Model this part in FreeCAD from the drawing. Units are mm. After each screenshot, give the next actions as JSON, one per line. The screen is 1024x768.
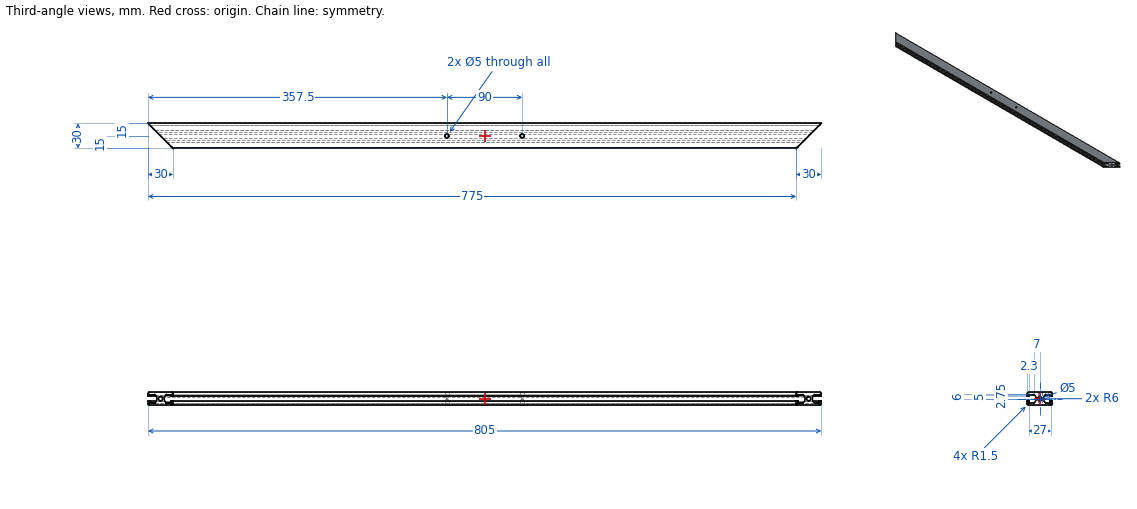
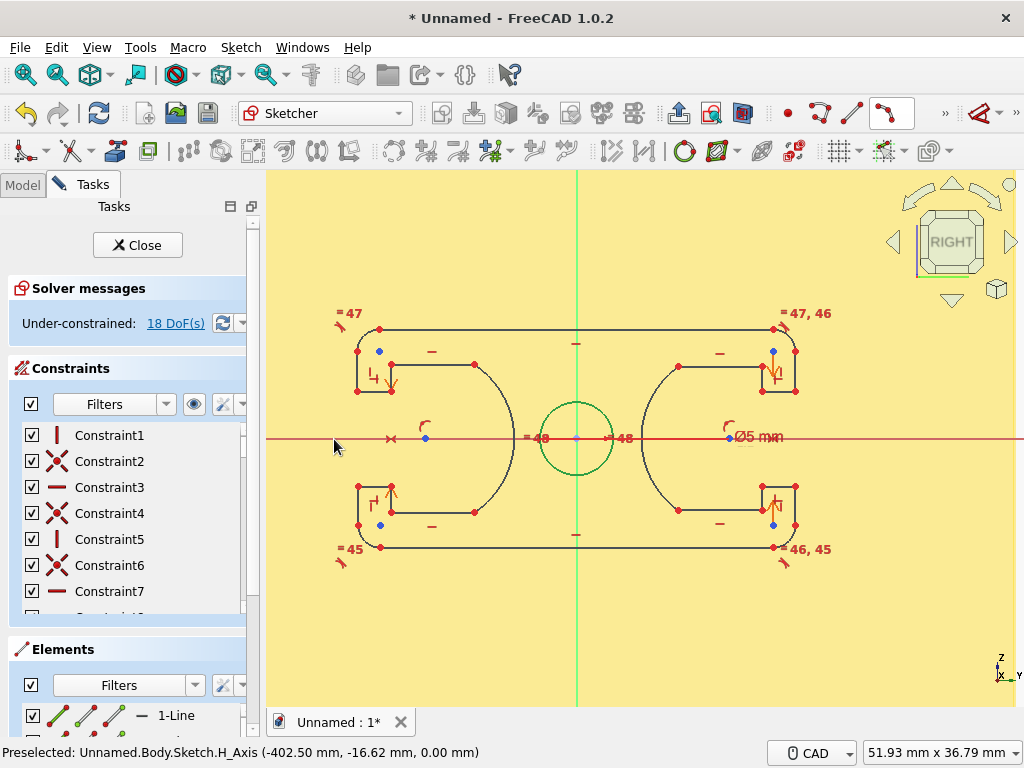
{"action": "left_click", "coordinate": [357, 392]}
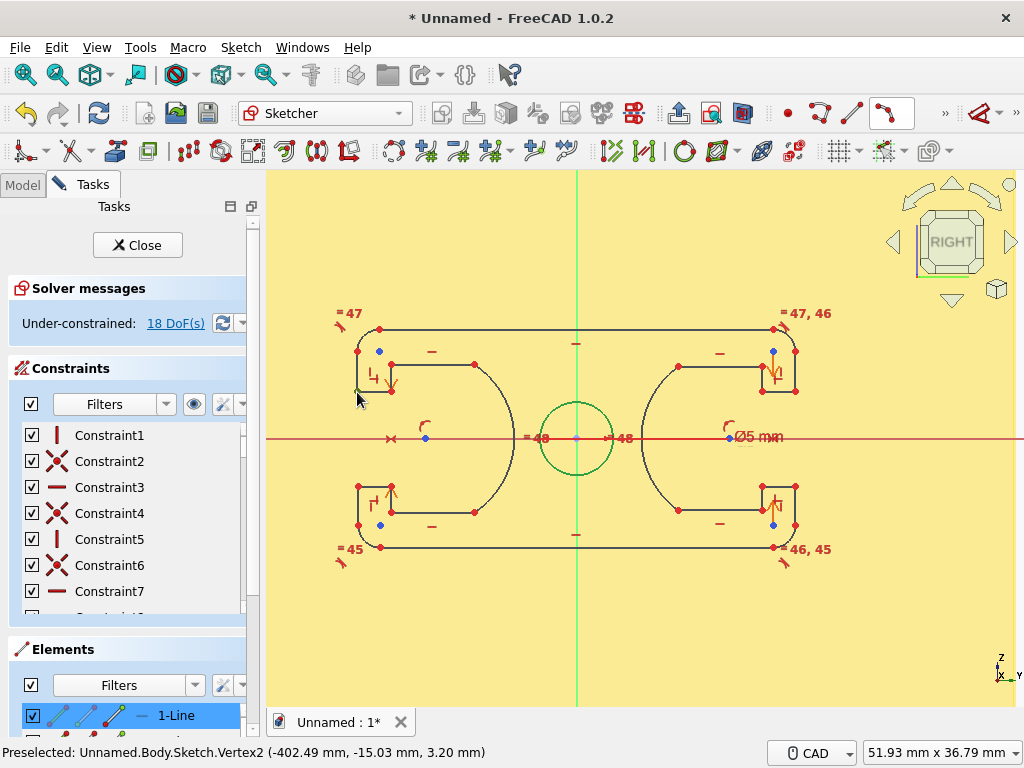
{"action": "left_click", "coordinate": [358, 487]}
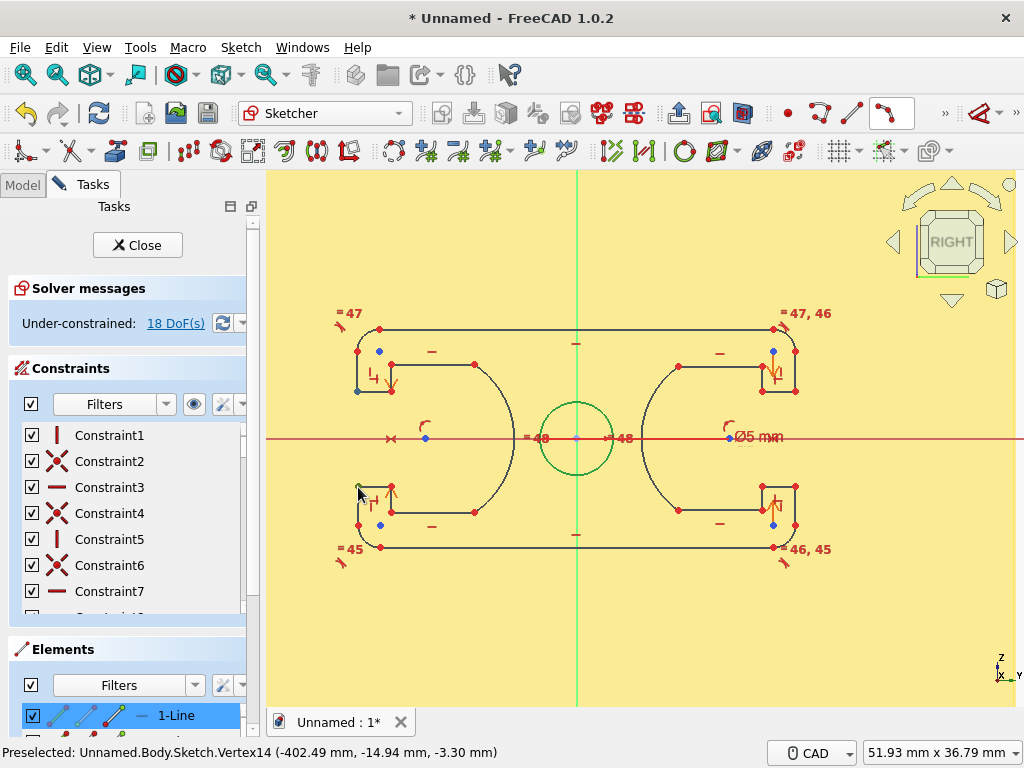
{"action": "left_click", "coordinate": [334, 439]}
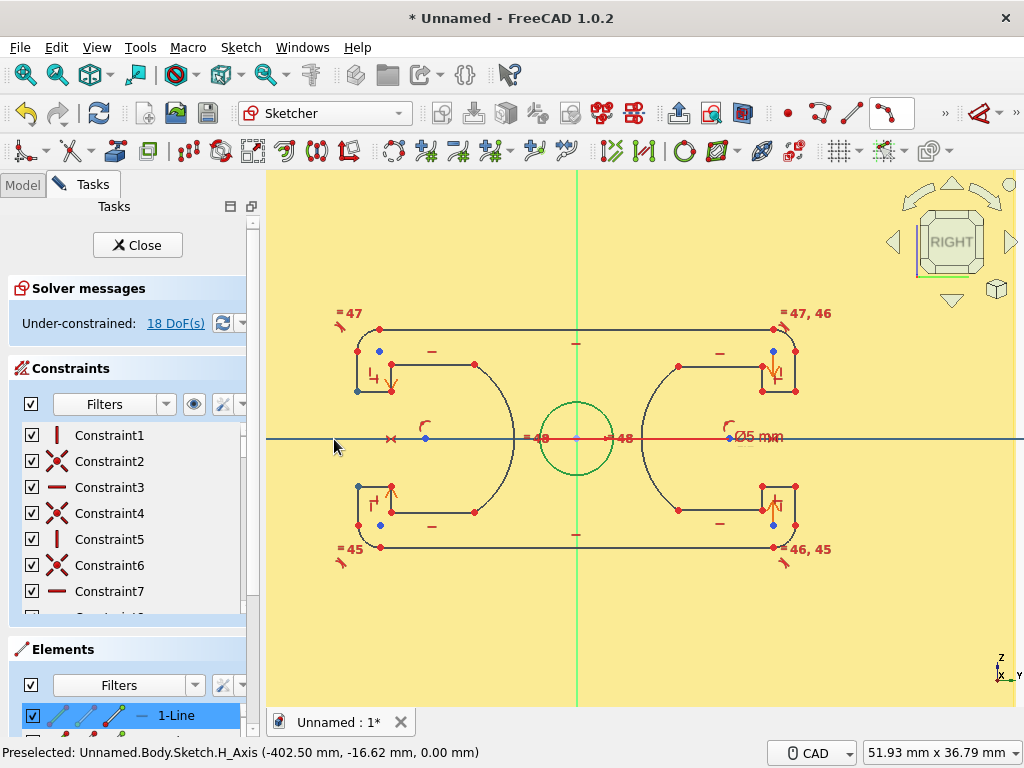
{"action": "key", "text": "s"}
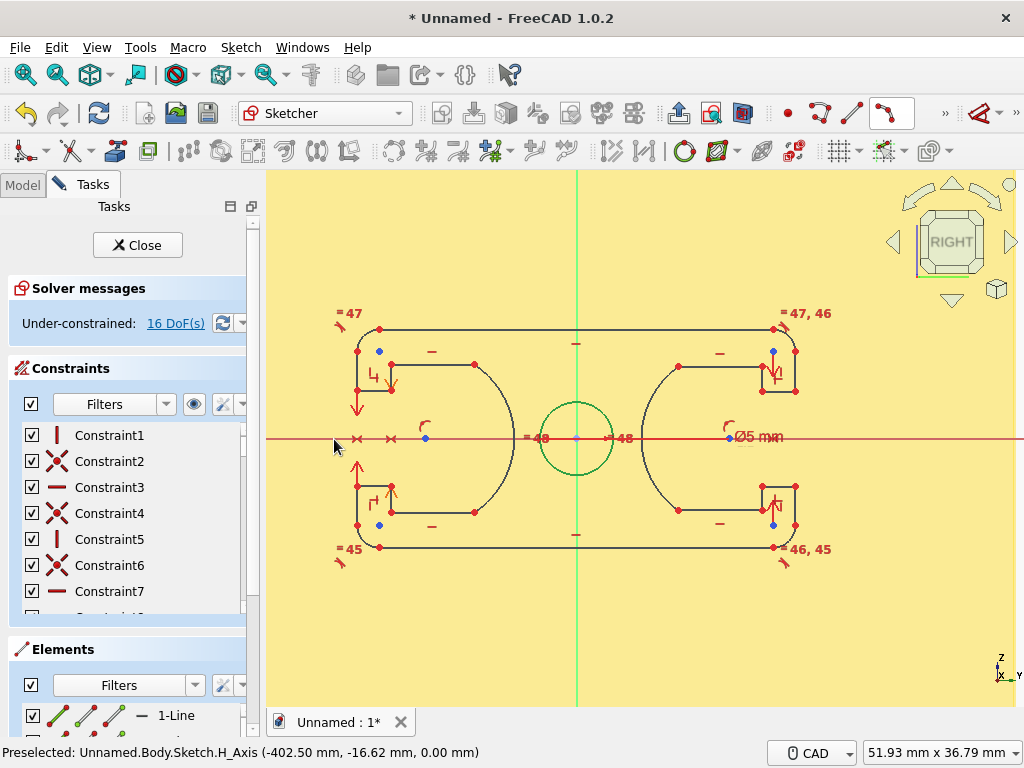
{"action": "left_click", "coordinate": [357, 486]}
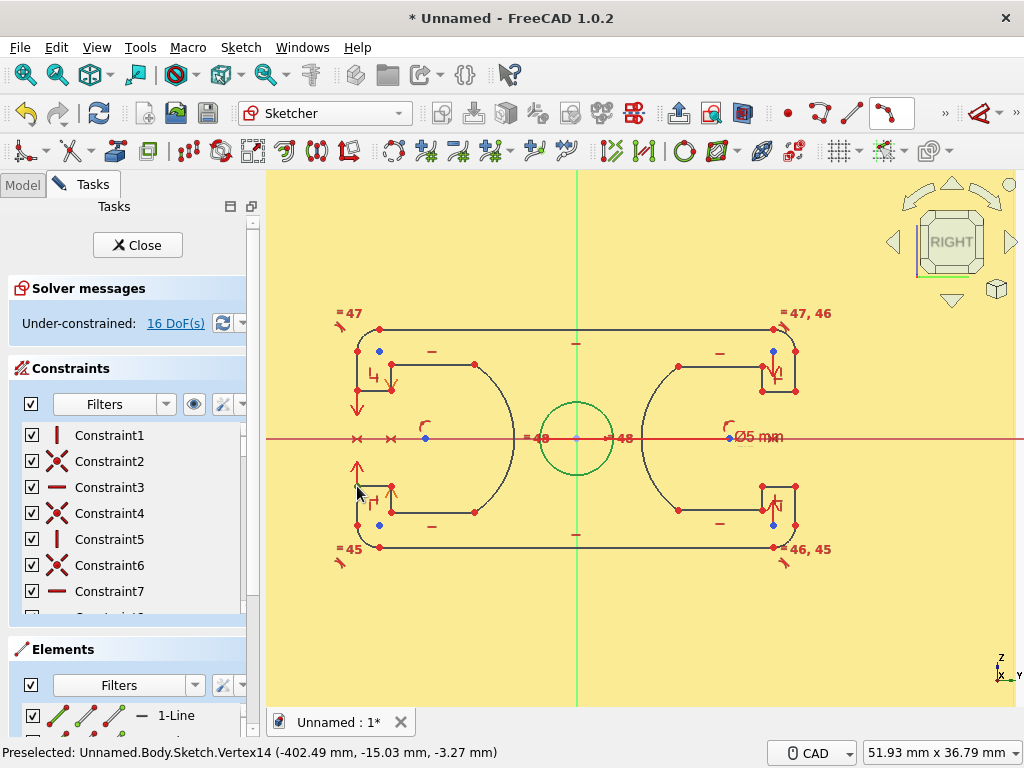
{"action": "left_click", "coordinate": [795, 487]}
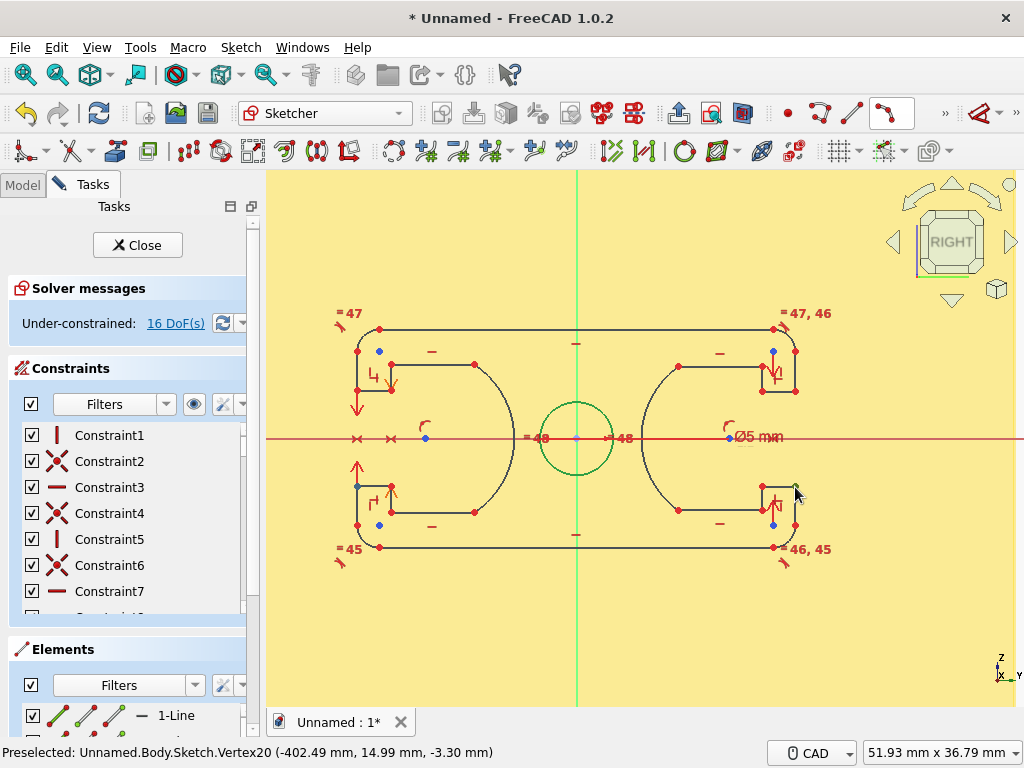
{"action": "left_click", "coordinate": [577, 645]}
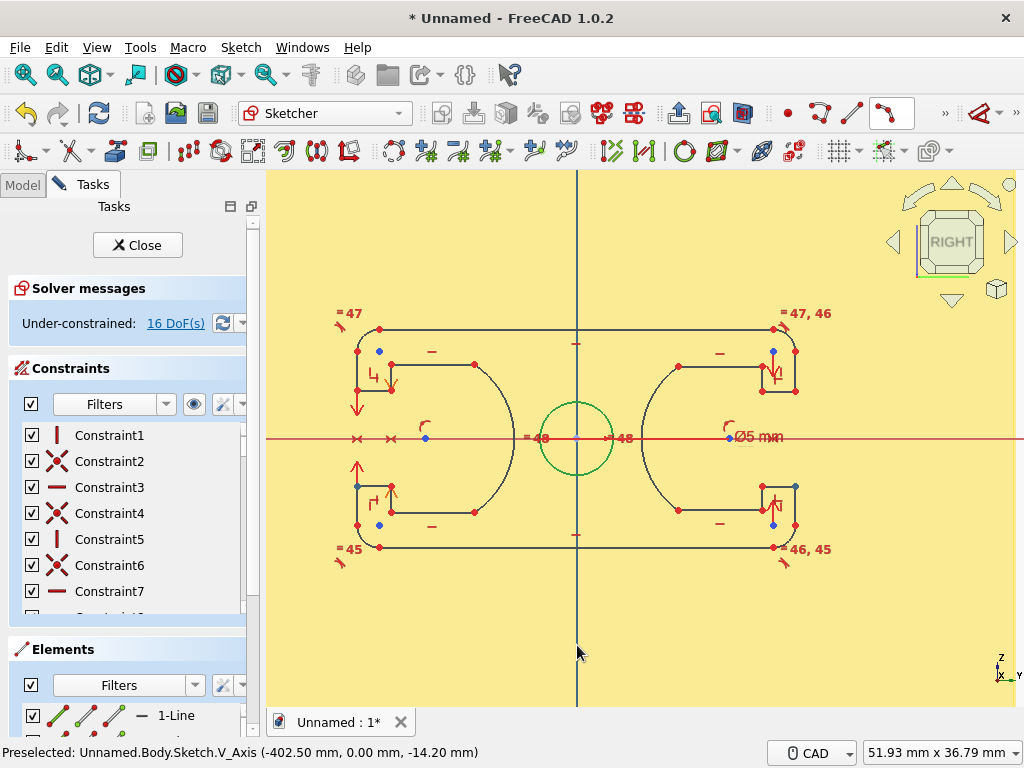
{"action": "key", "text": "s"}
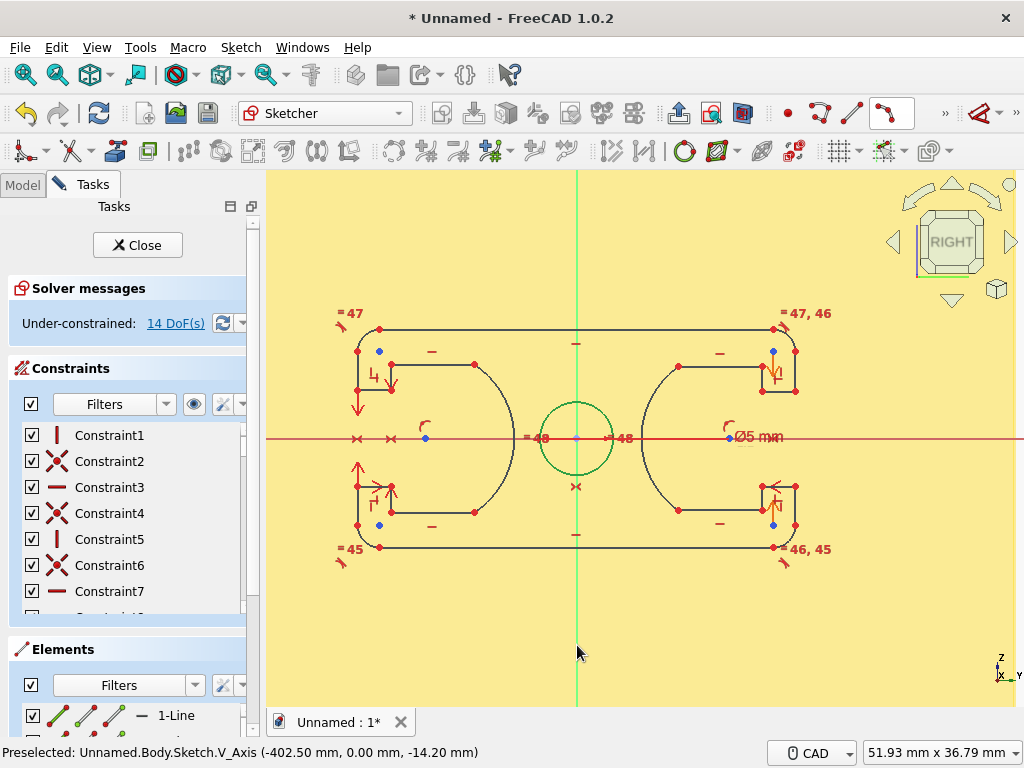
{"action": "left_click", "coordinate": [391, 513]}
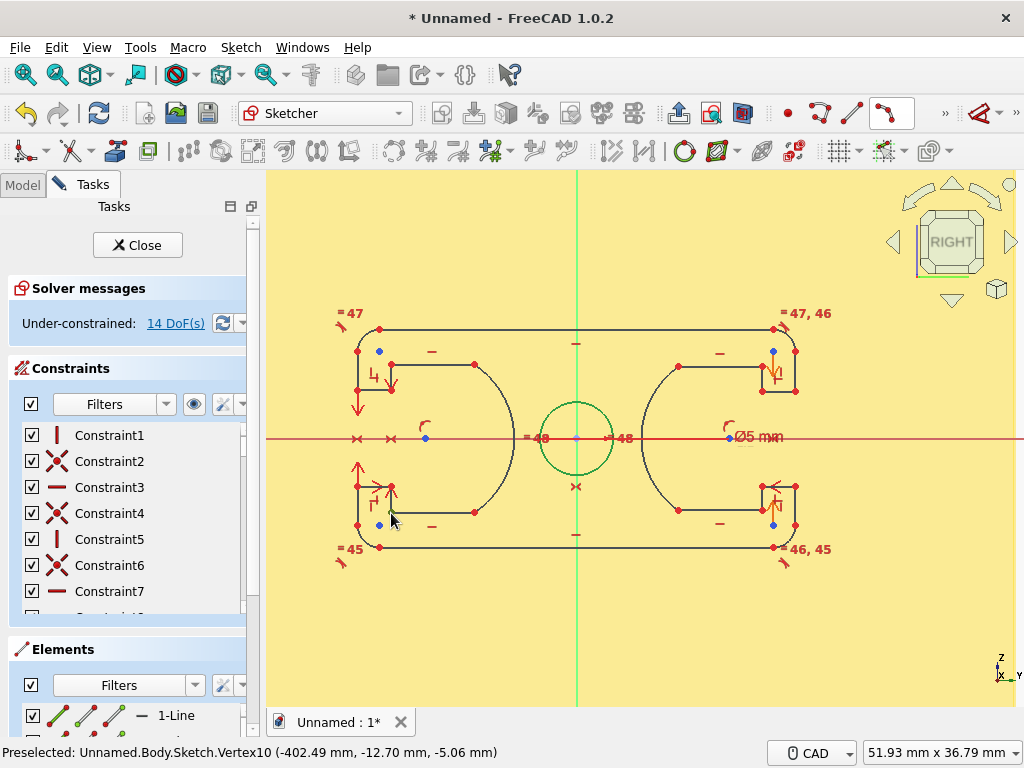
{"action": "left_click", "coordinate": [762, 510]}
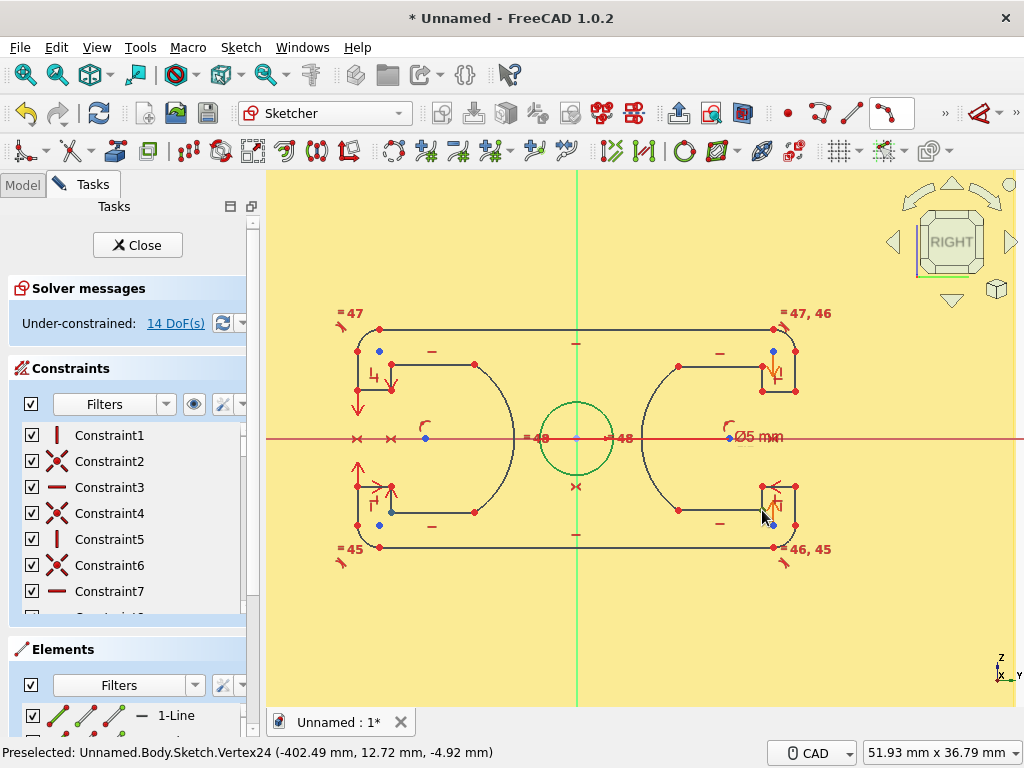
{"action": "left_click", "coordinate": [577, 645]}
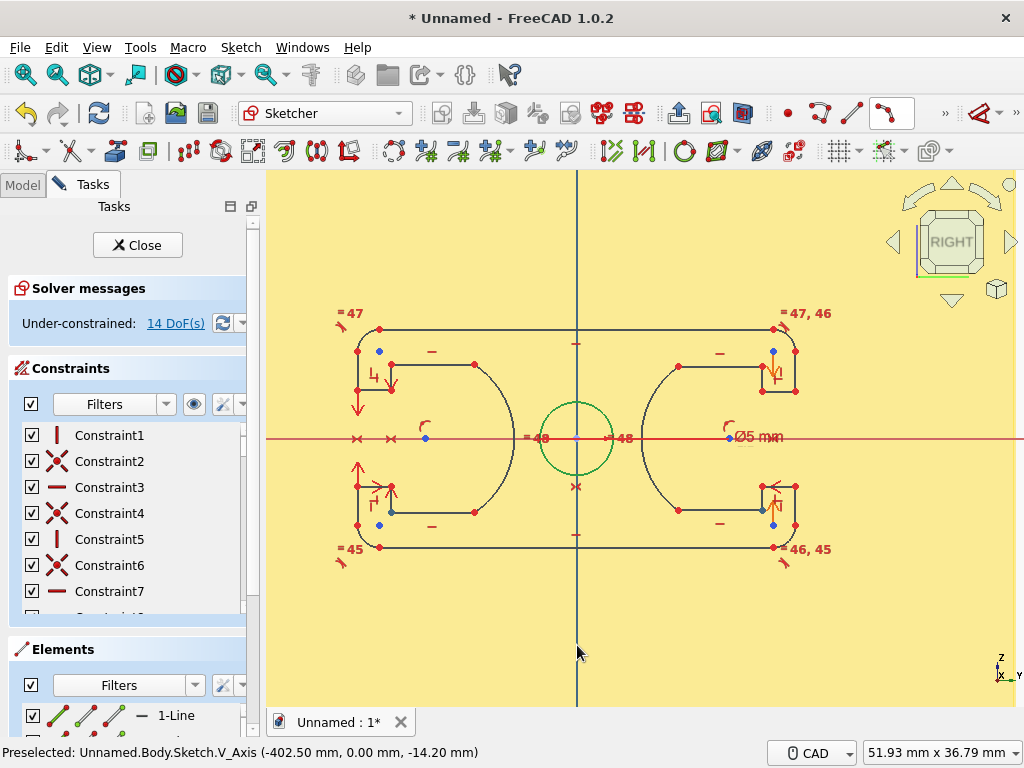
{"action": "key", "text": "s"}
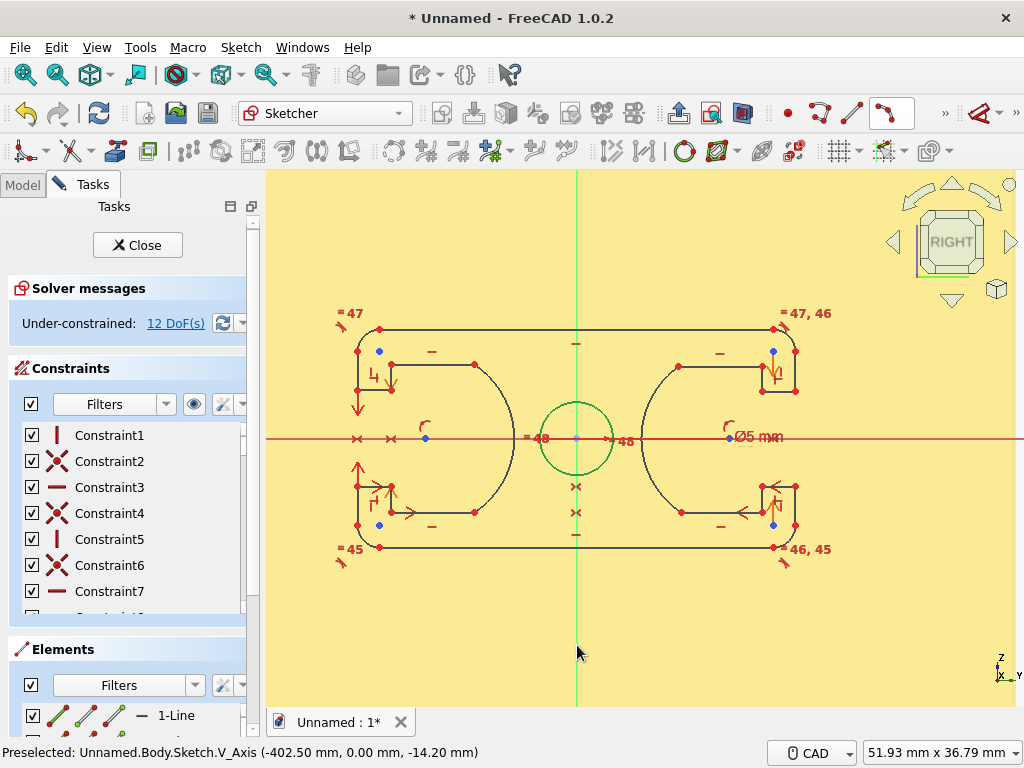
{"action": "left_click", "coordinate": [474, 365]}